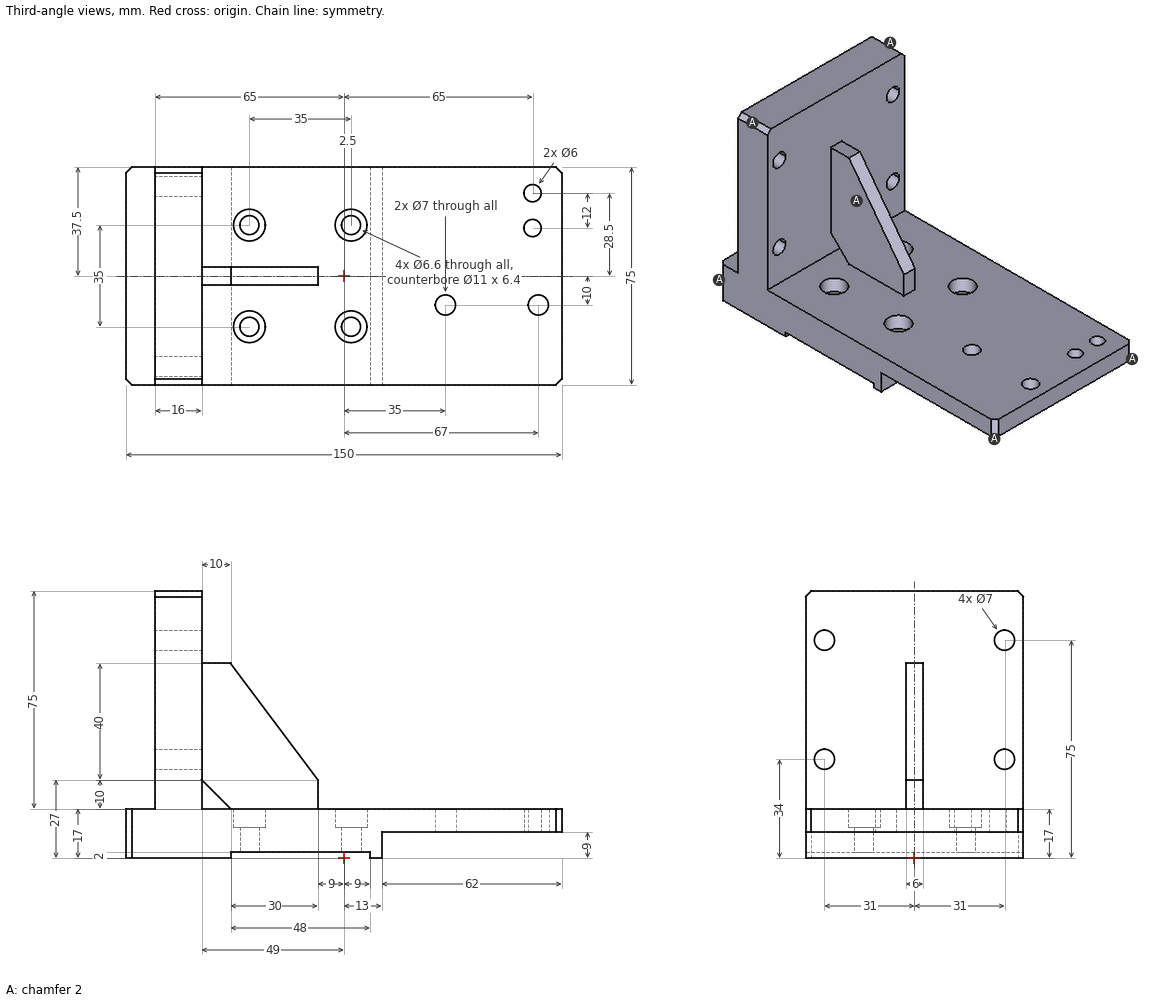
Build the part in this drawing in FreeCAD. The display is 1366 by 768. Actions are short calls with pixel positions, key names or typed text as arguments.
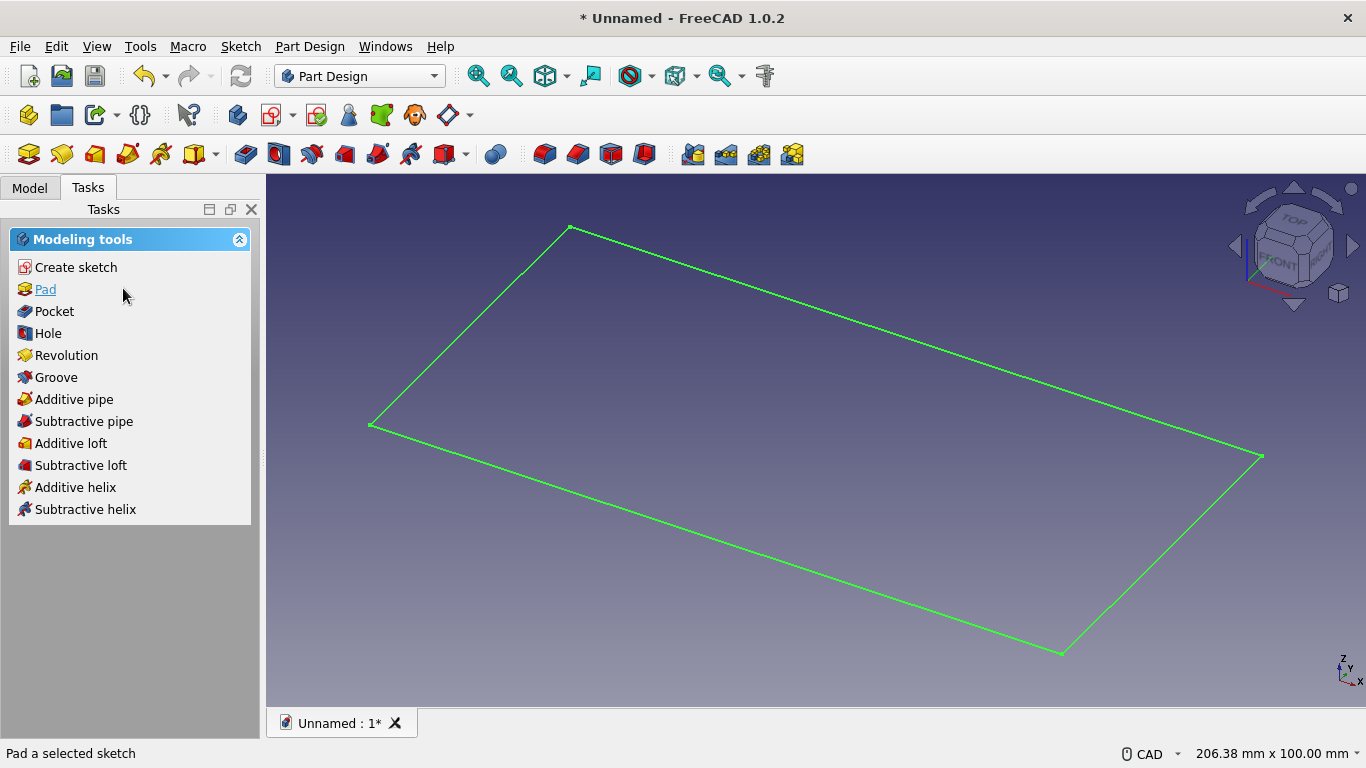
click(29, 154)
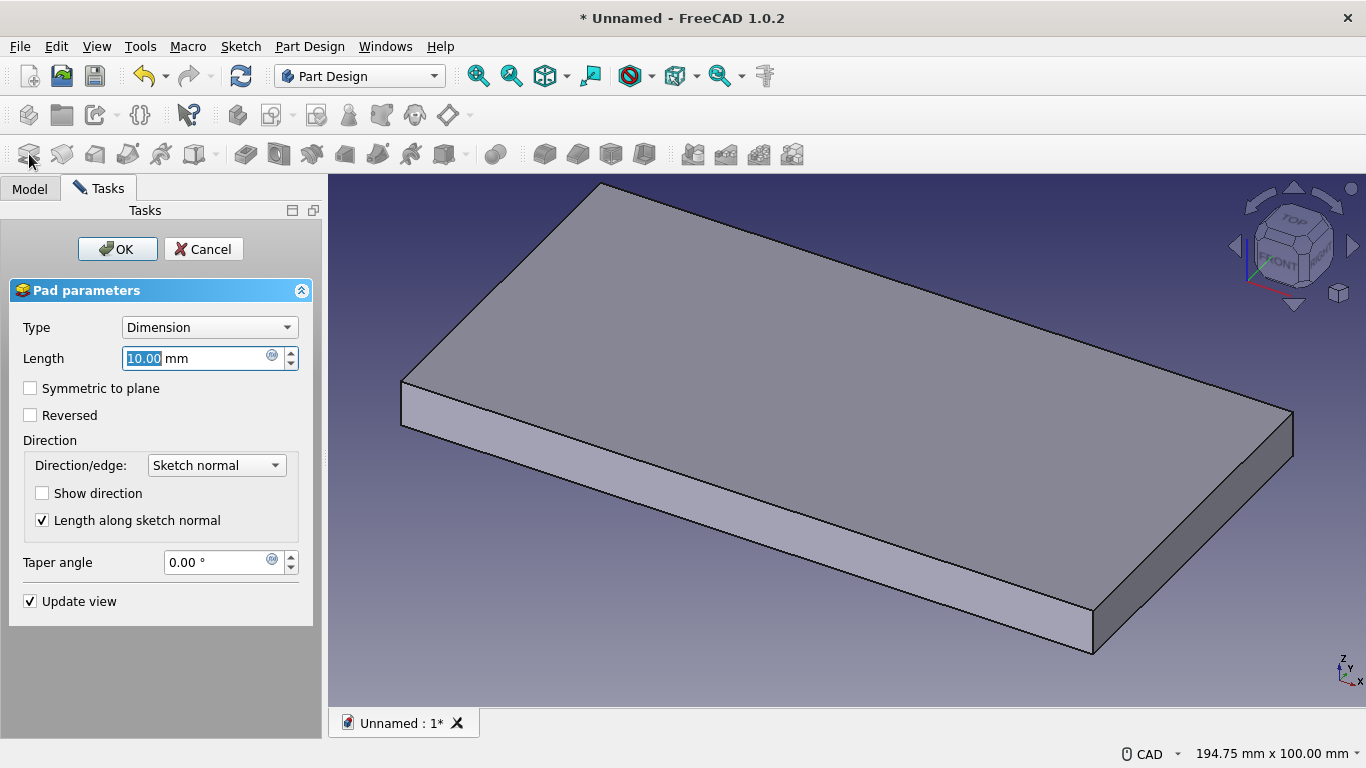
text(17)
key(Tab)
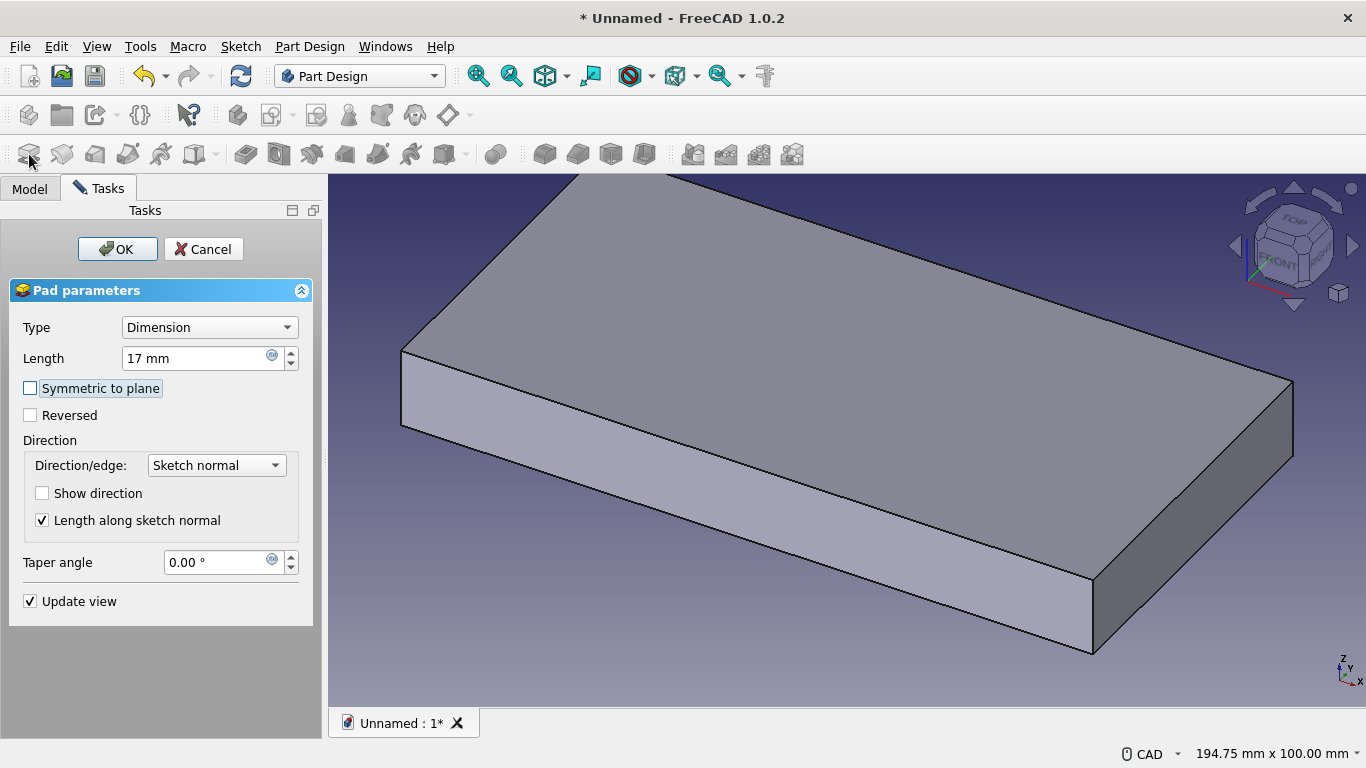
click(118, 249)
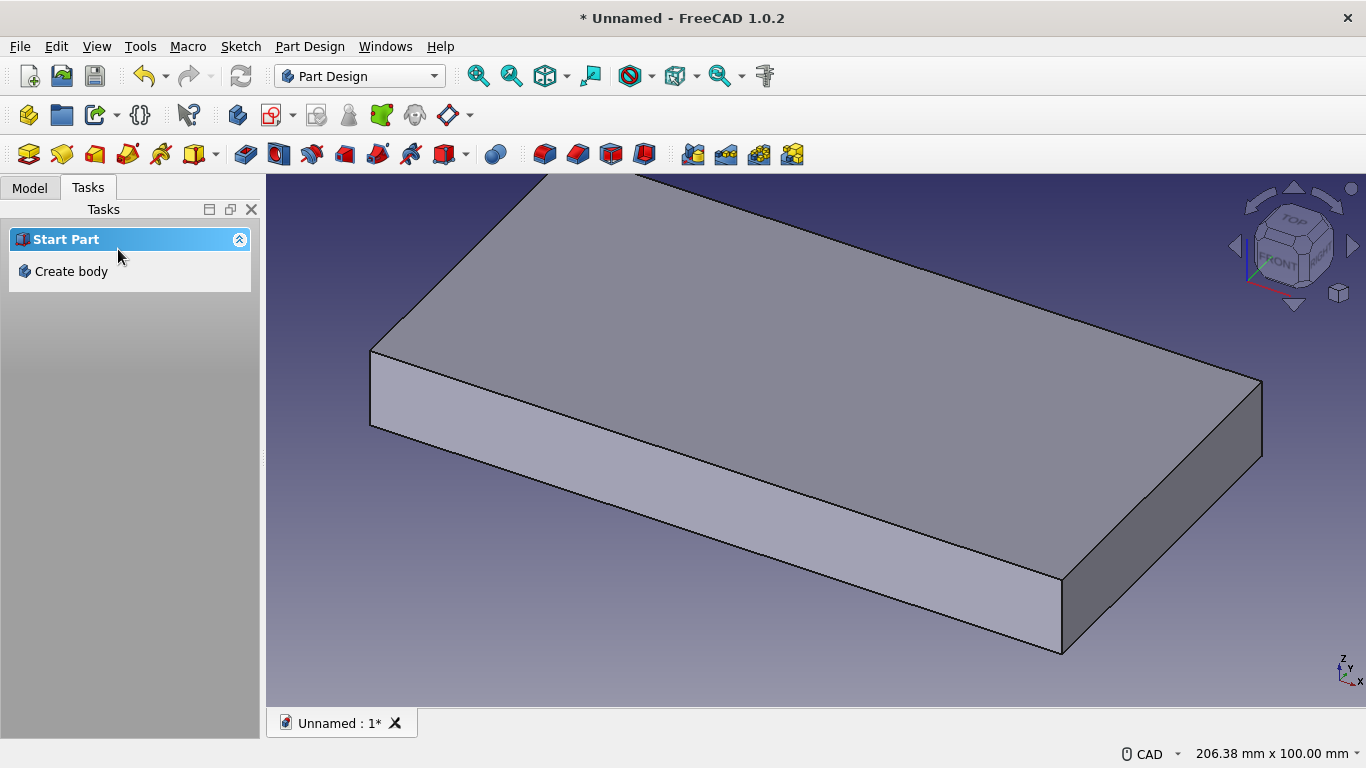
click(479, 76)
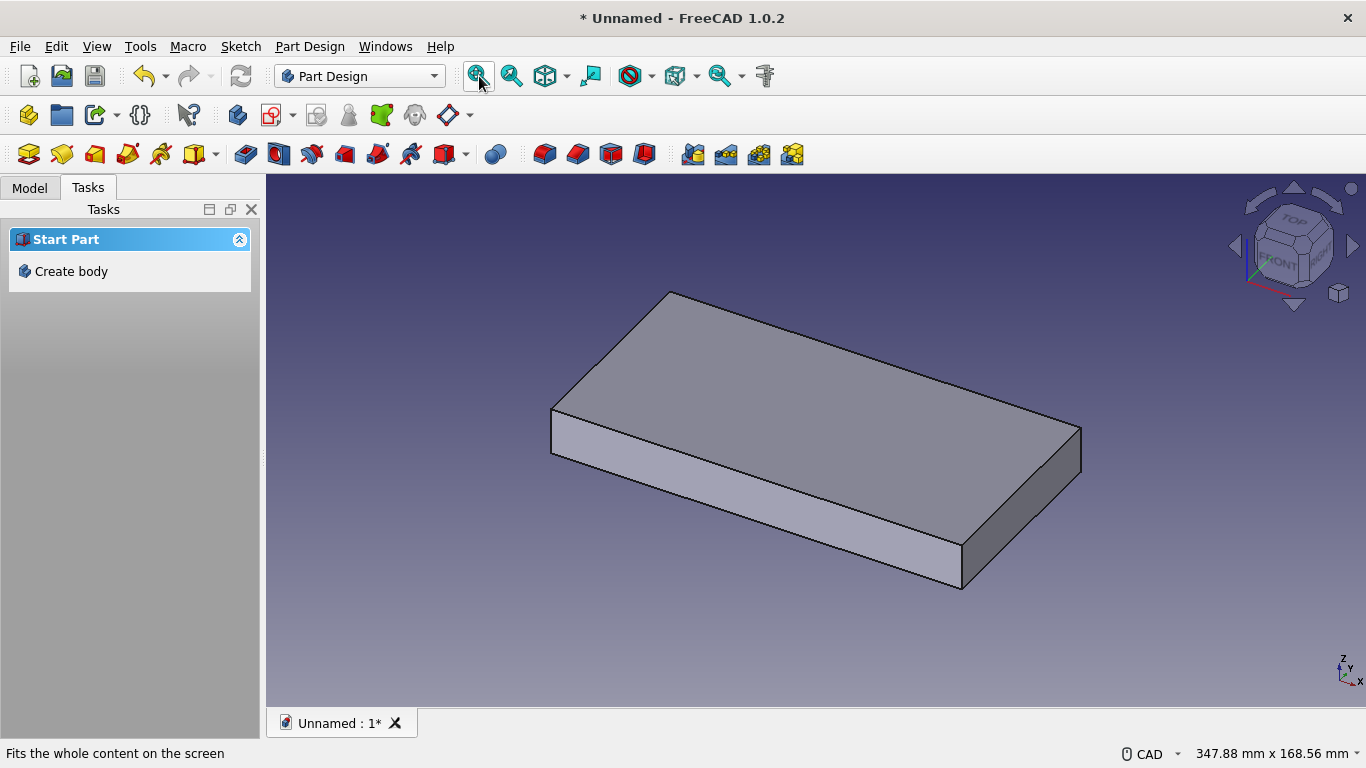
click(875, 437)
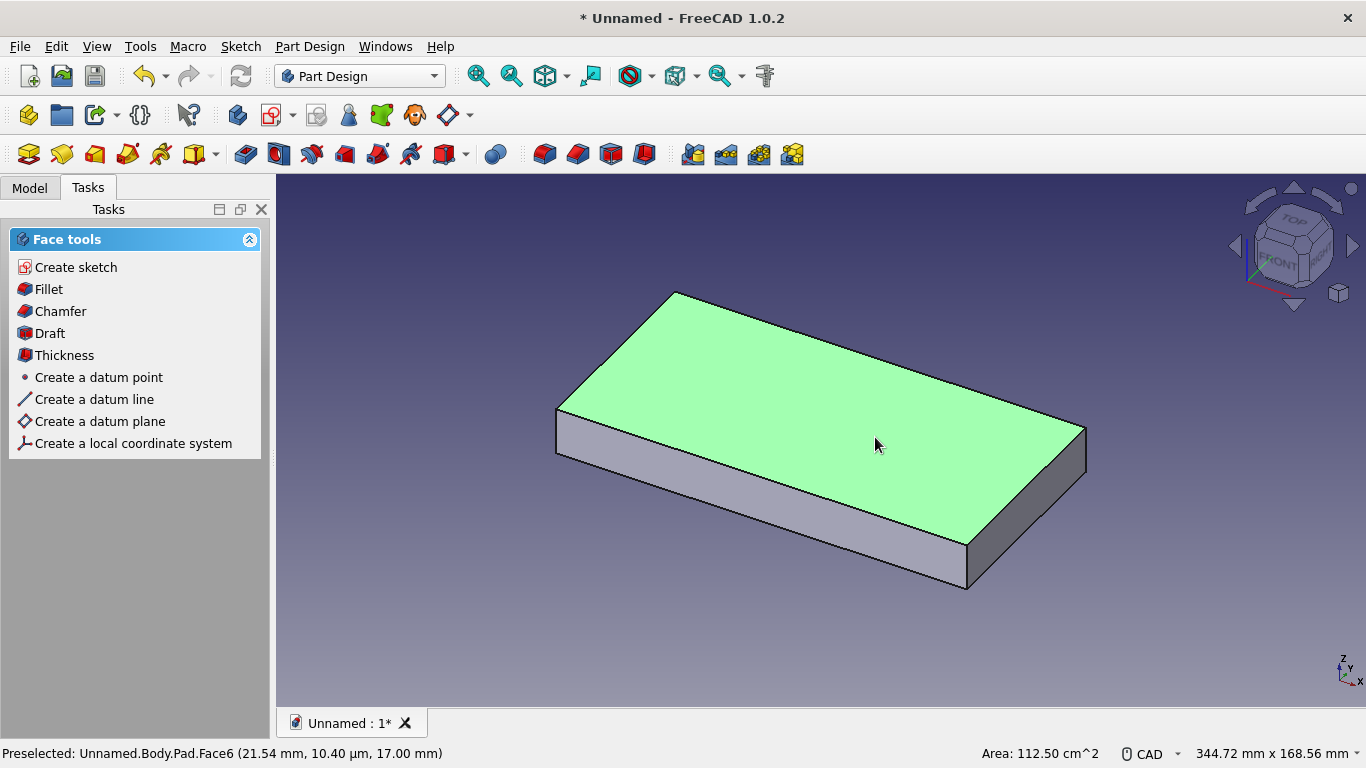
click(270, 116)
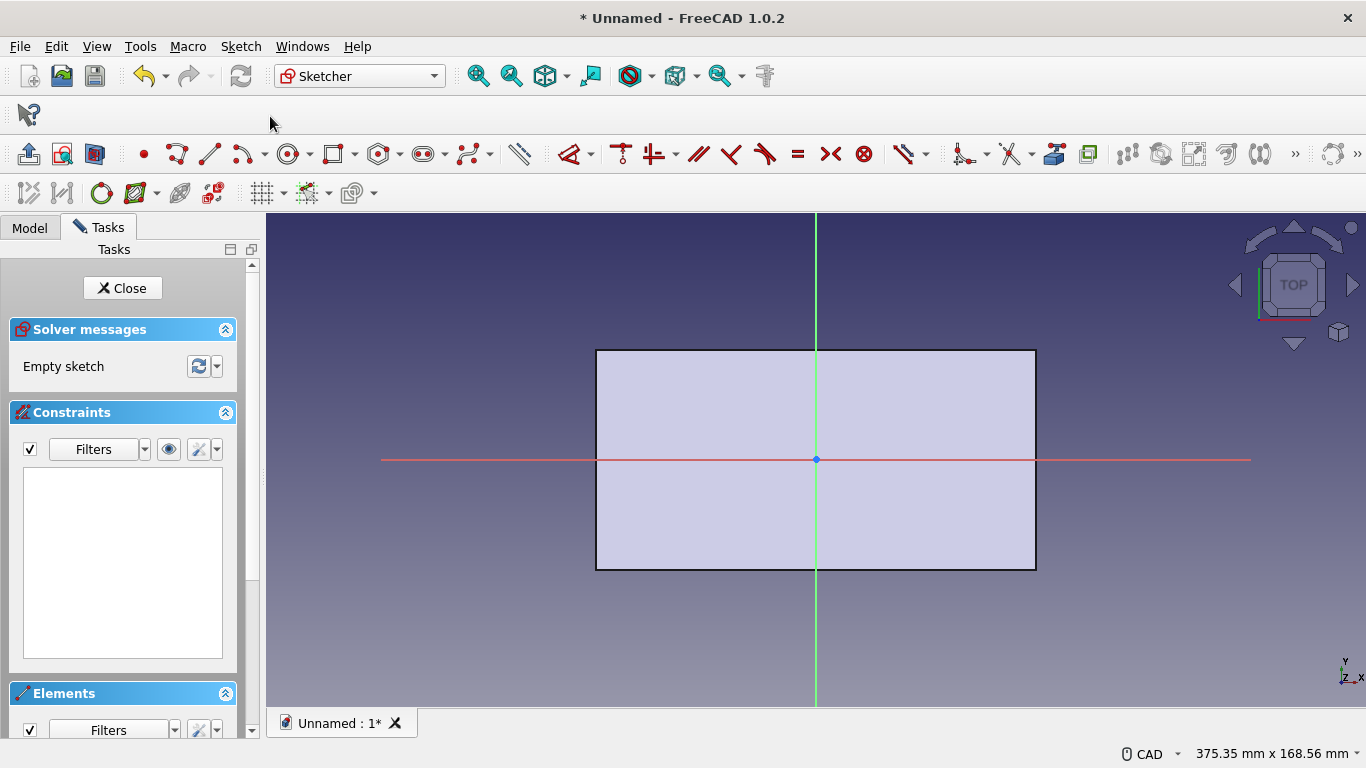
scroll(786, 460, up, 5)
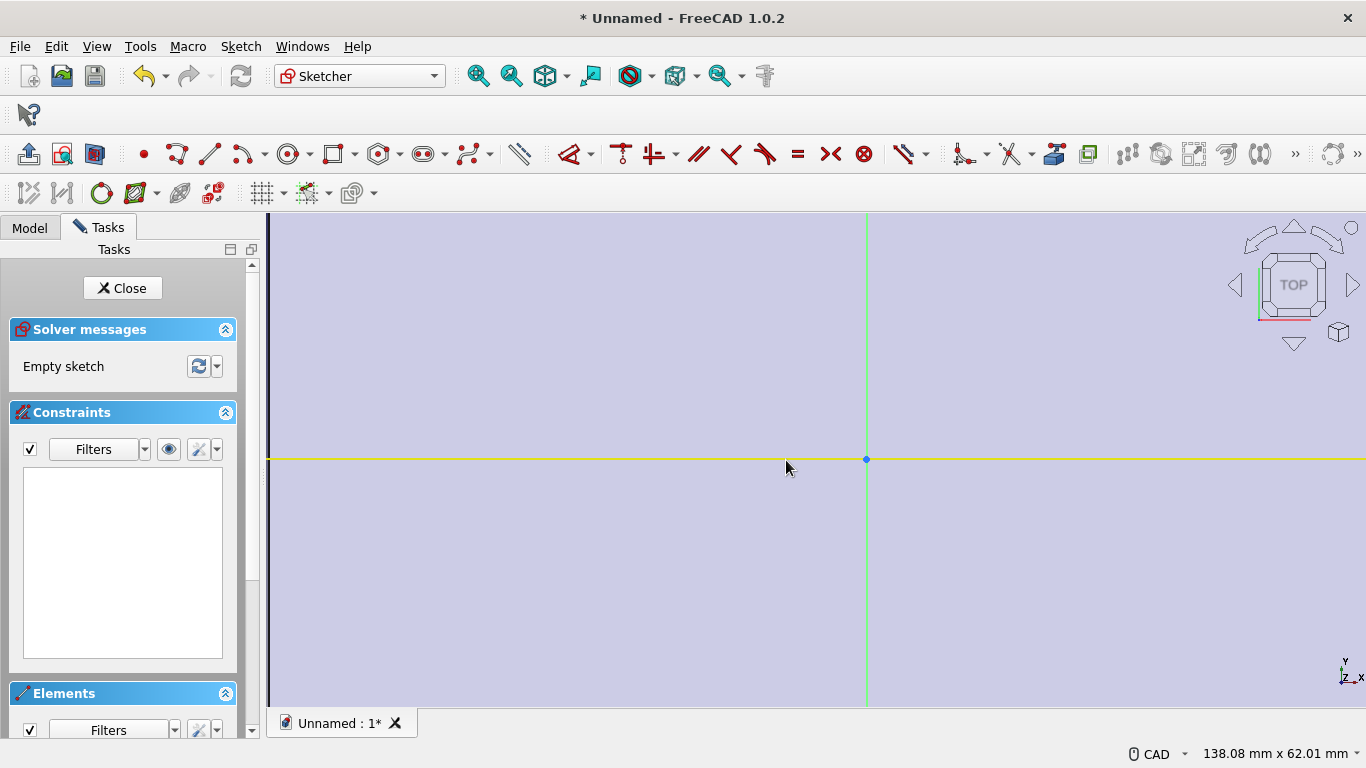
click(288, 154)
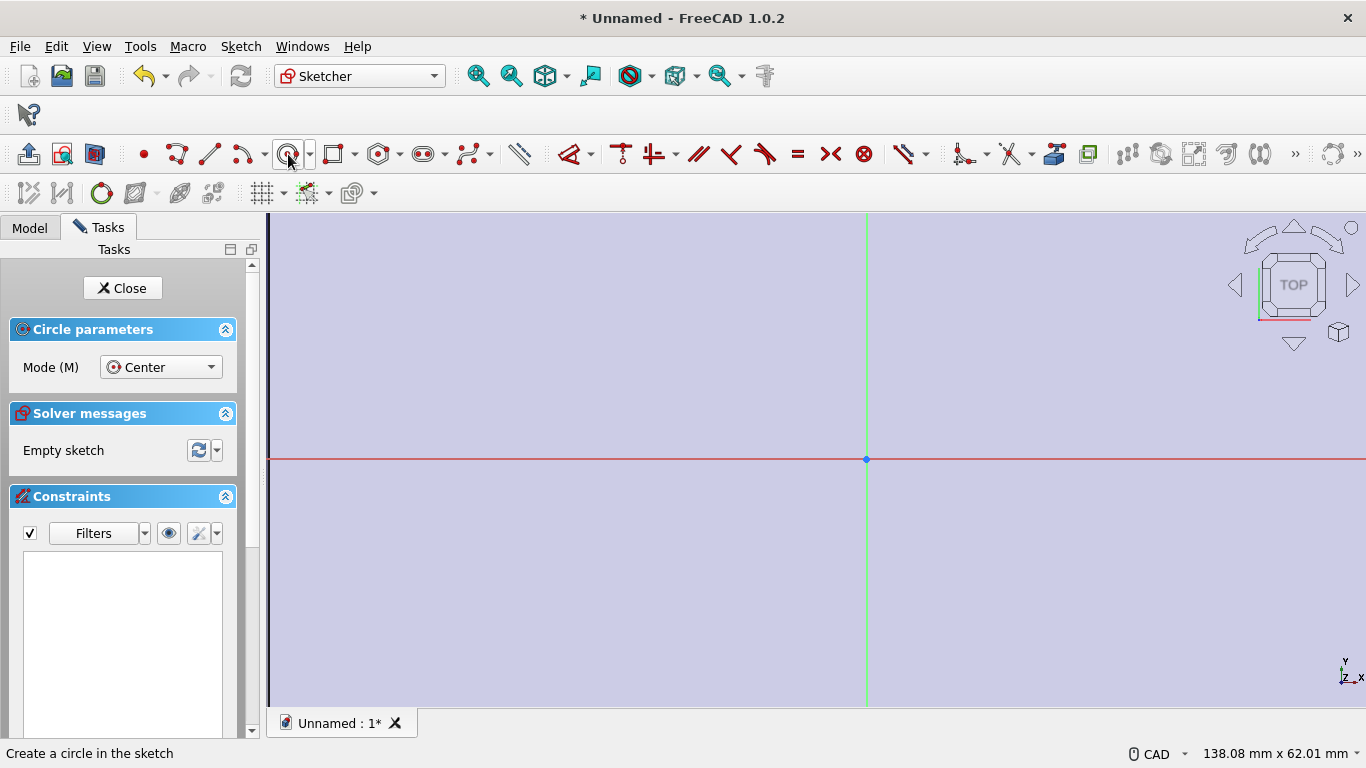
click(887, 320)
move(905, 301)